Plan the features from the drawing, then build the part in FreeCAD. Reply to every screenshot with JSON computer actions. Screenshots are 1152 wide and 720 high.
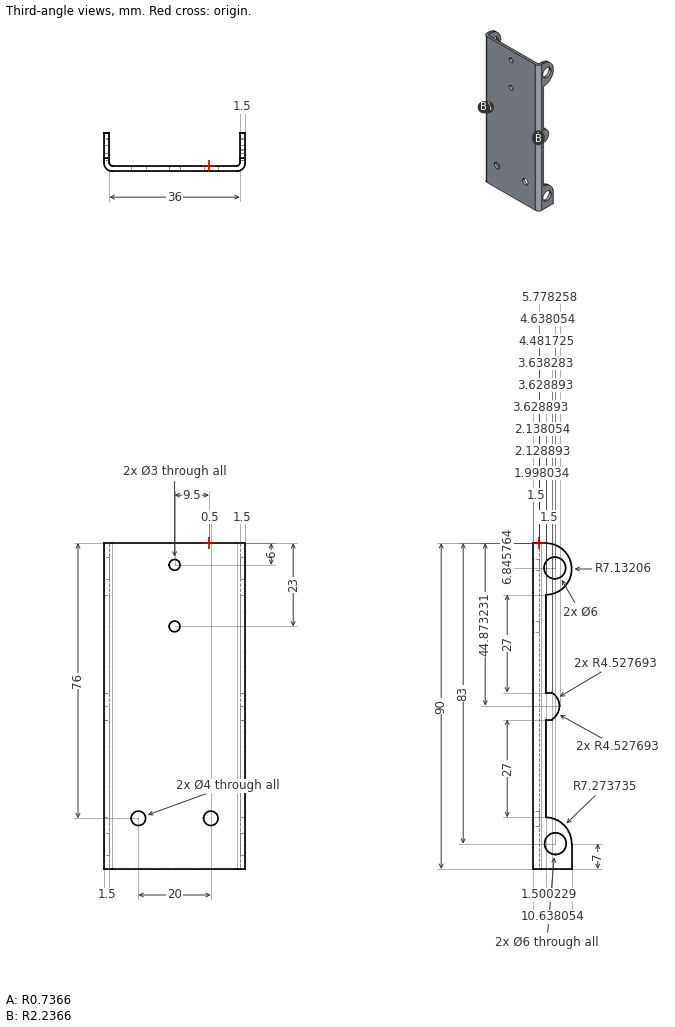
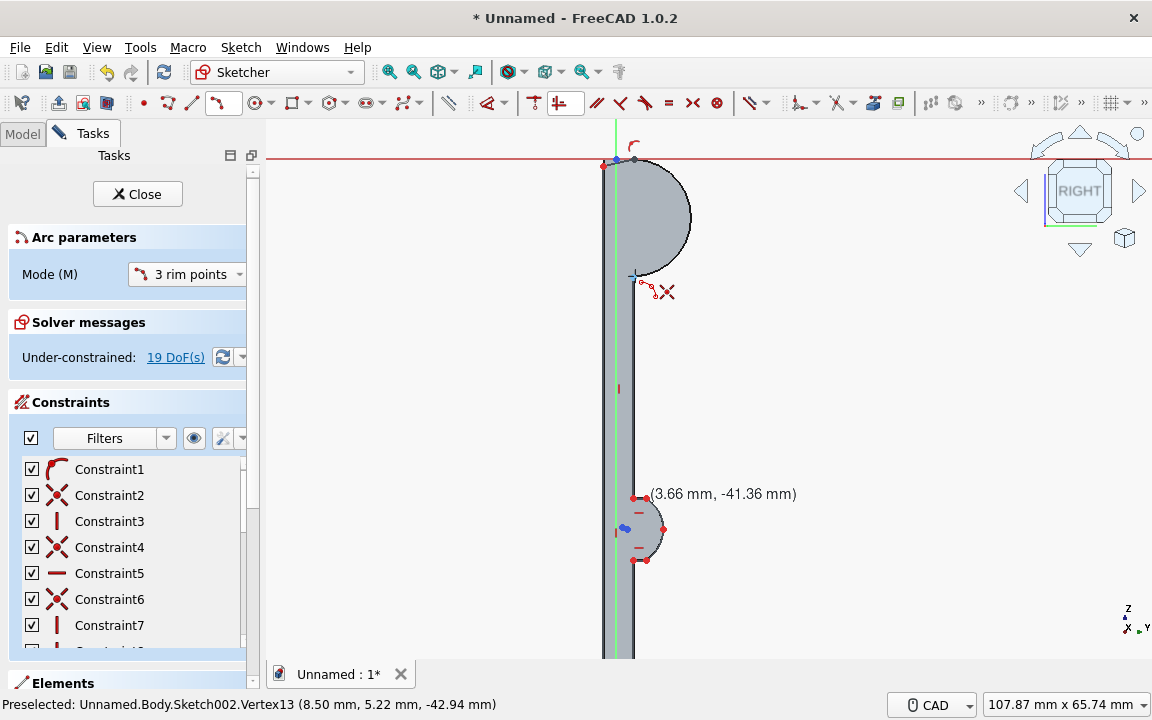
{"action": "left_click", "coordinate": [633, 278]}
{"action": "left_click", "coordinate": [634, 159]}
{"action": "left_click", "coordinate": [691, 218]}
{"action": "key", "text": "Escape"}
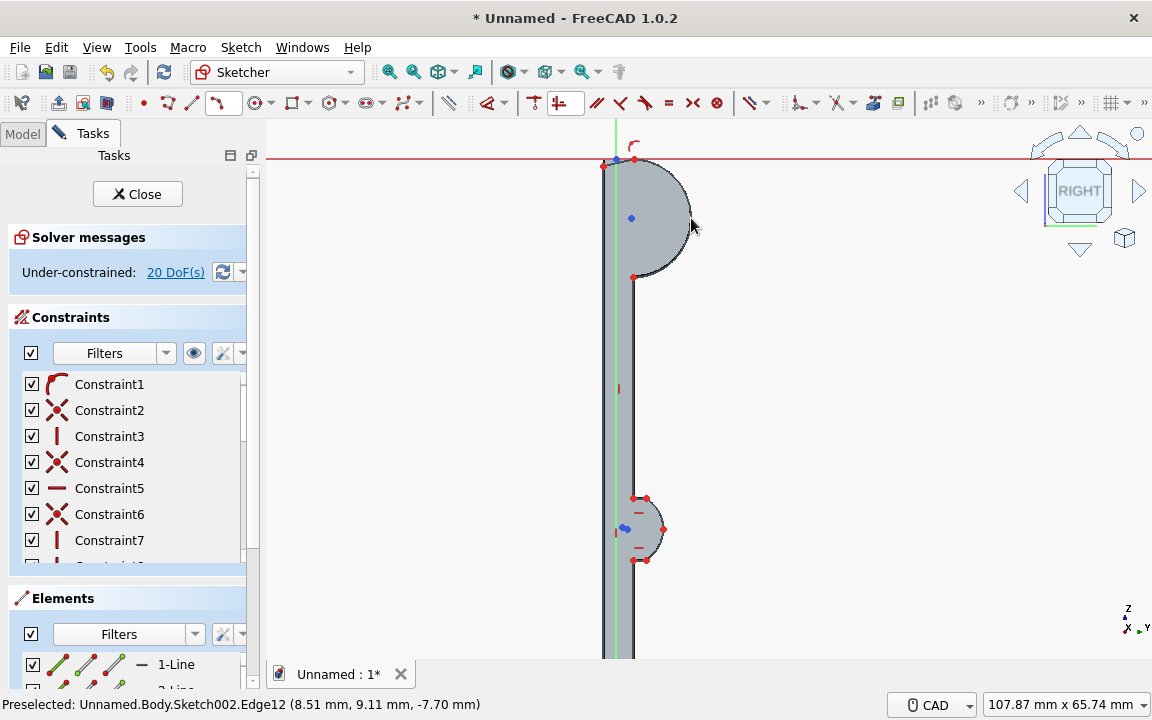
{"action": "scroll", "coordinate": [635, 275], "scroll_direction": "down", "scroll_amount": 4}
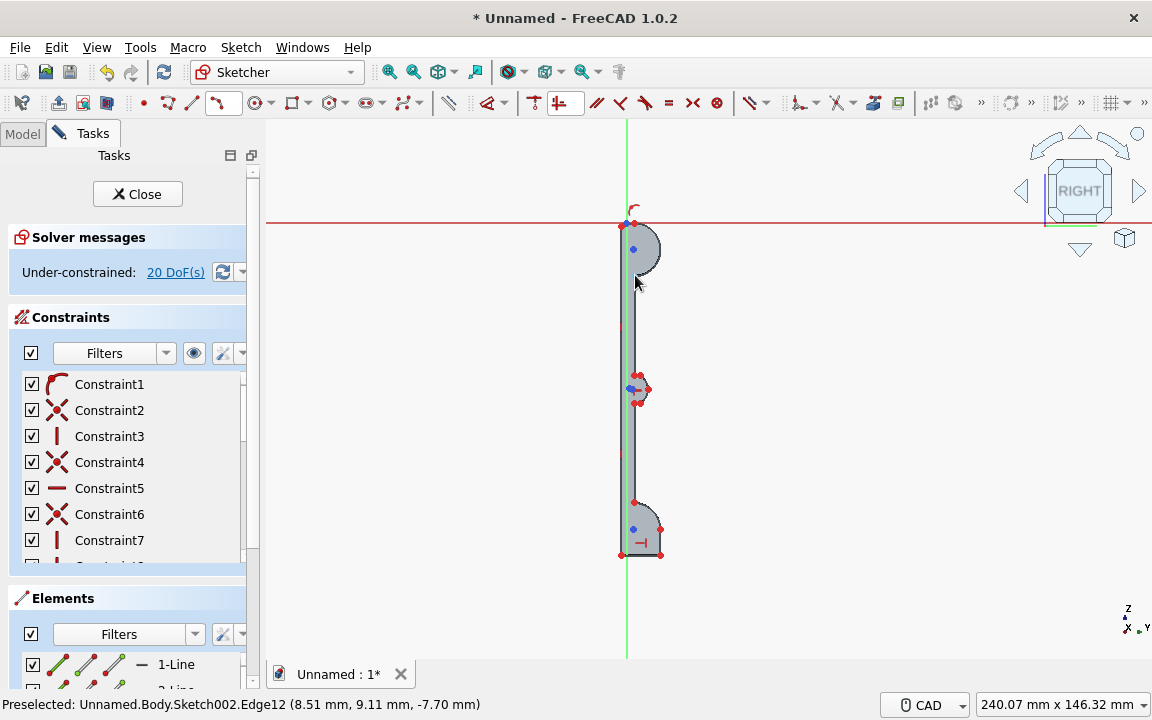
{"action": "scroll", "coordinate": [660, 548], "scroll_direction": "up", "scroll_amount": 3}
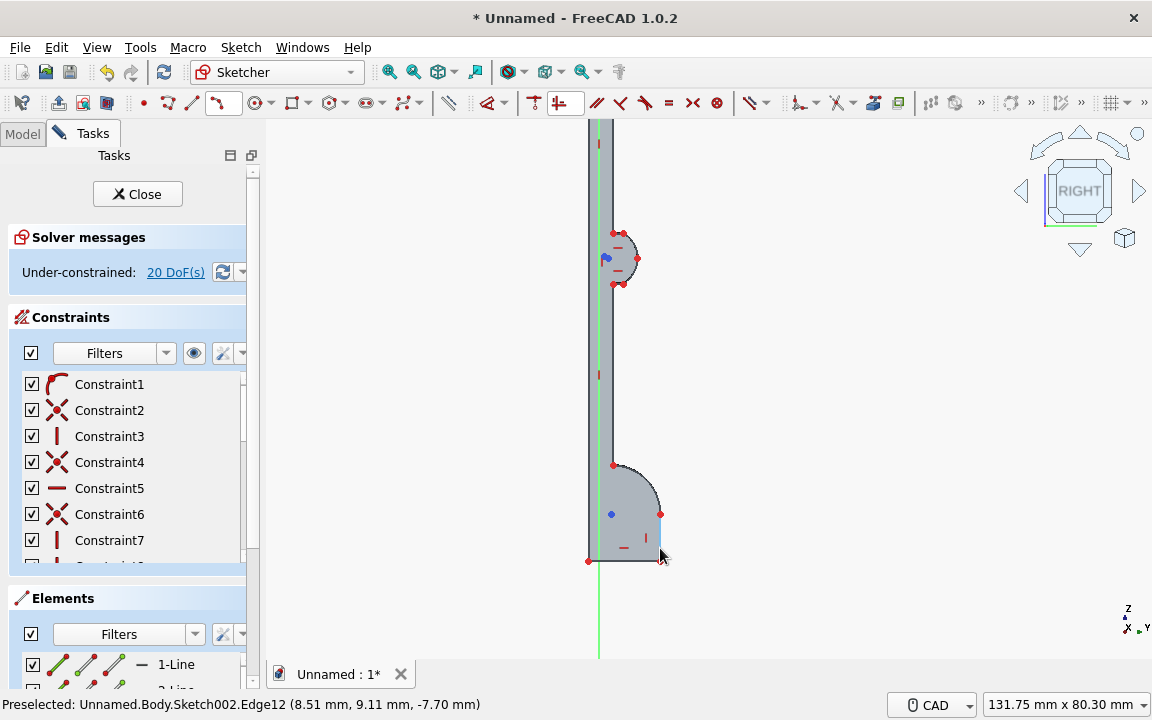
{"action": "left_click", "coordinate": [660, 547]}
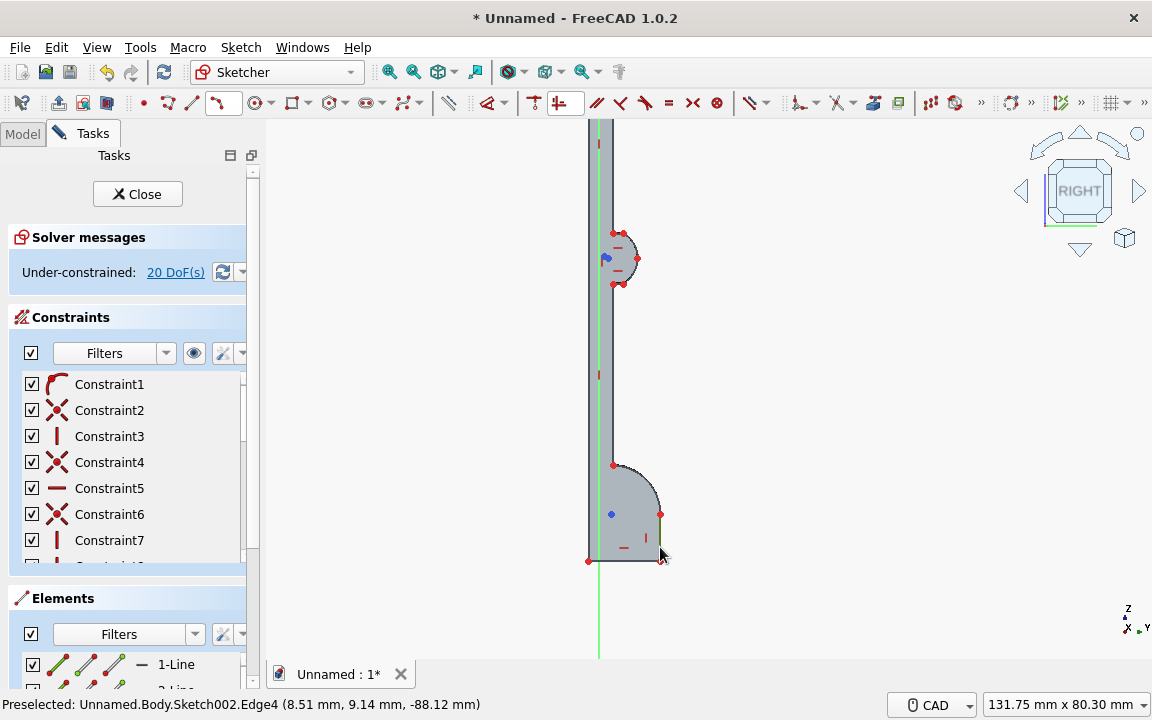
{"action": "left_click", "coordinate": [655, 492]}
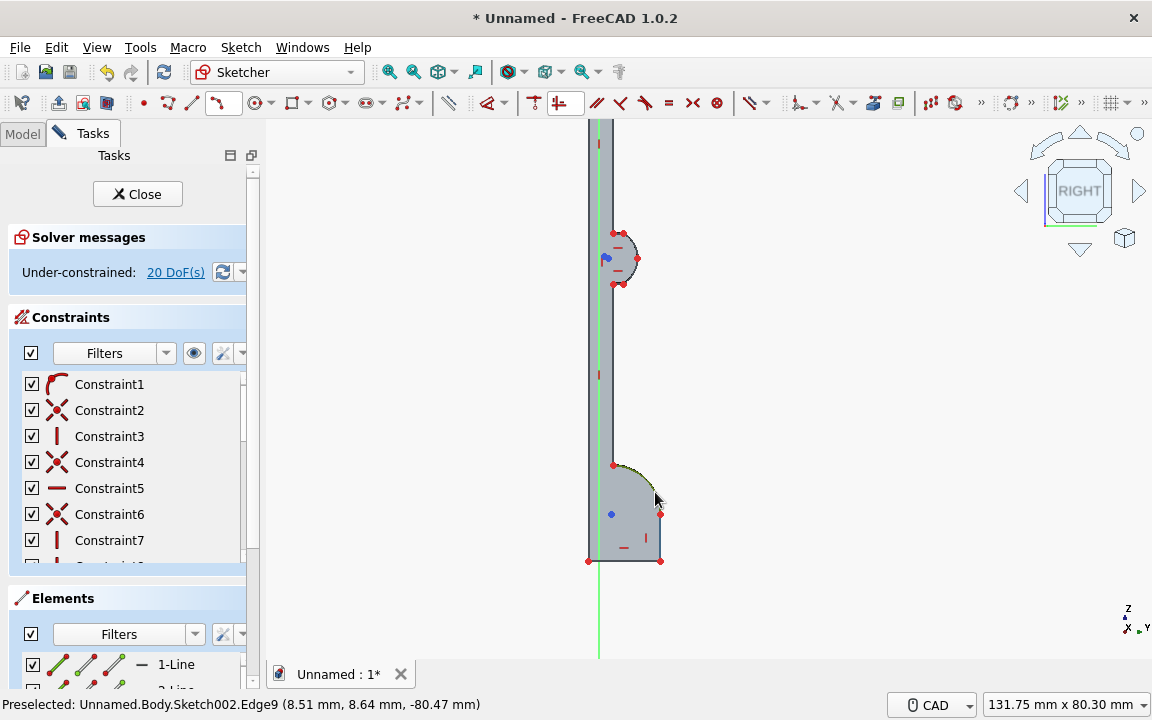
{"action": "key", "text": "t"}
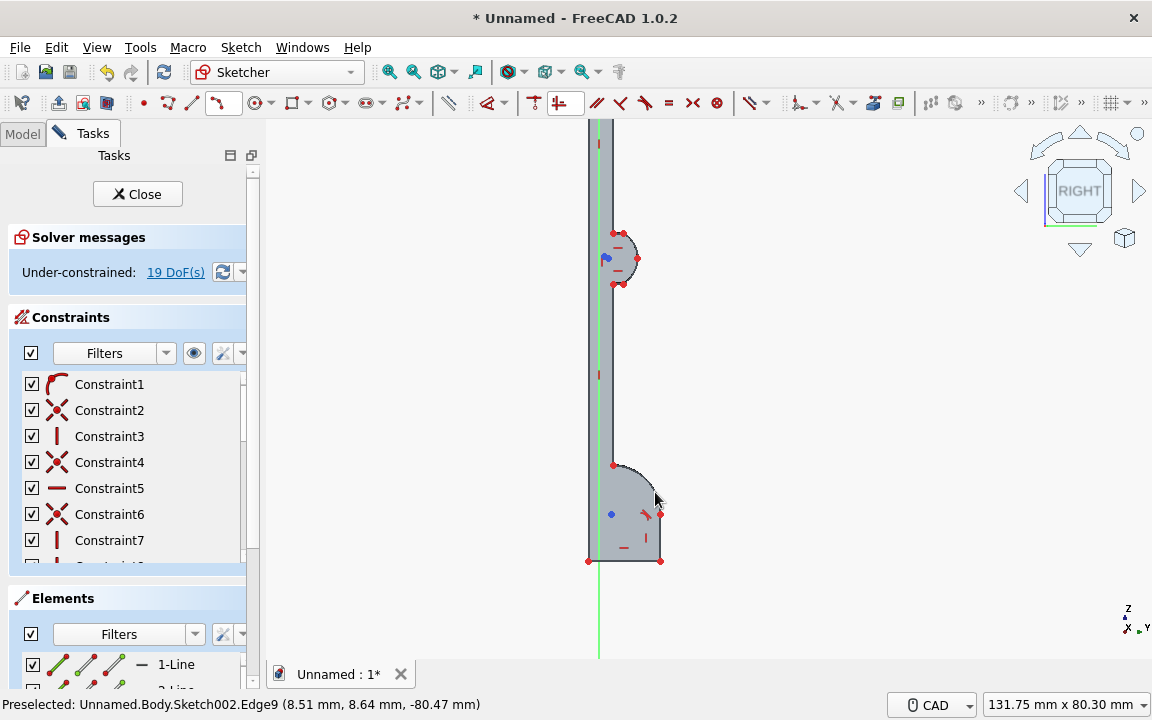
{"action": "scroll", "coordinate": [660, 548], "scroll_direction": "down", "scroll_amount": 3}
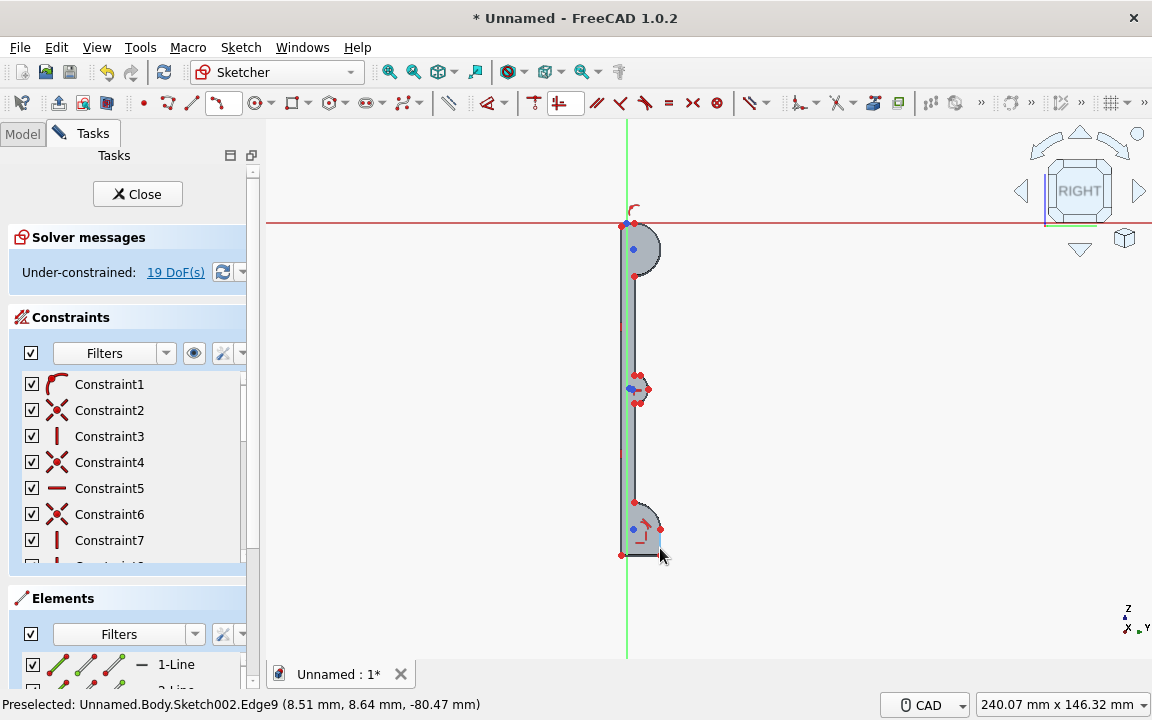
{"action": "scroll", "coordinate": [627, 225], "scroll_direction": "up", "scroll_amount": 5}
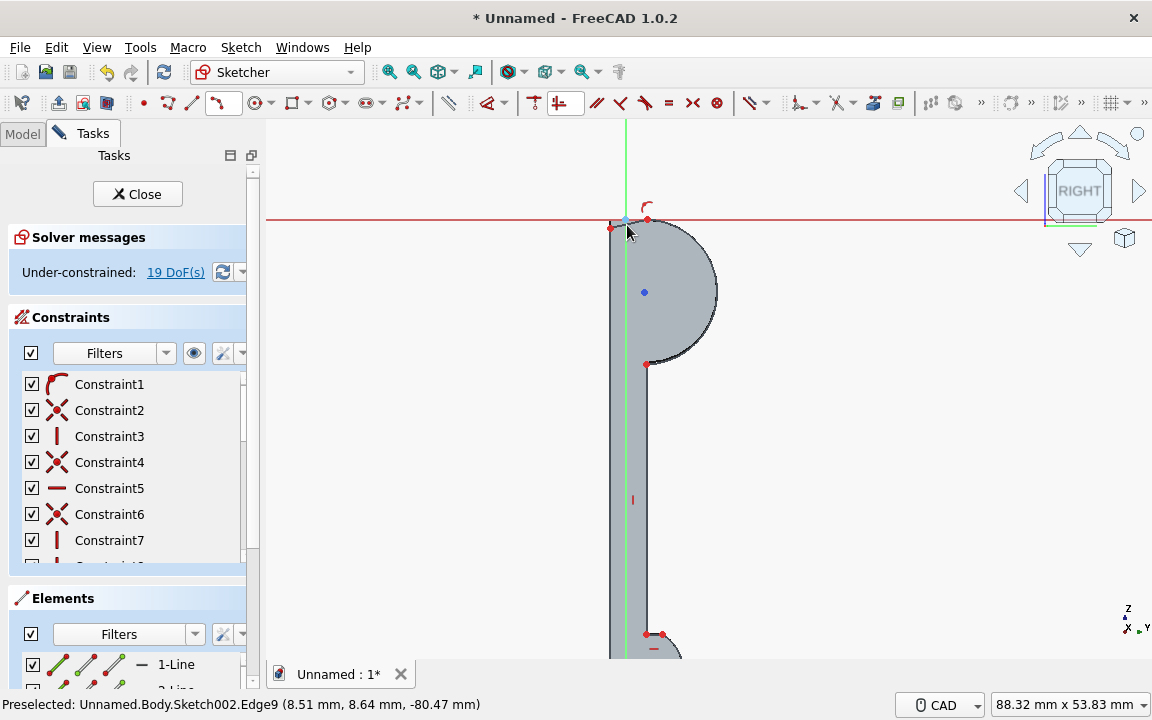
{"action": "left_click", "coordinate": [625, 225]}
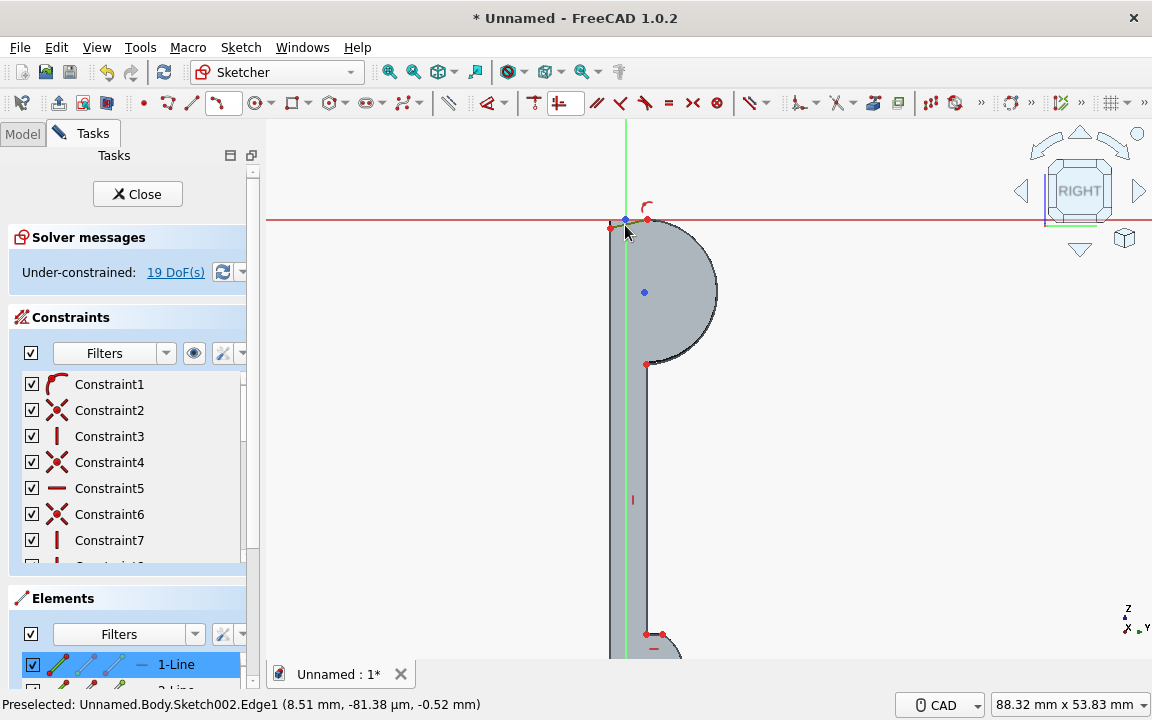
{"action": "key", "text": "h"}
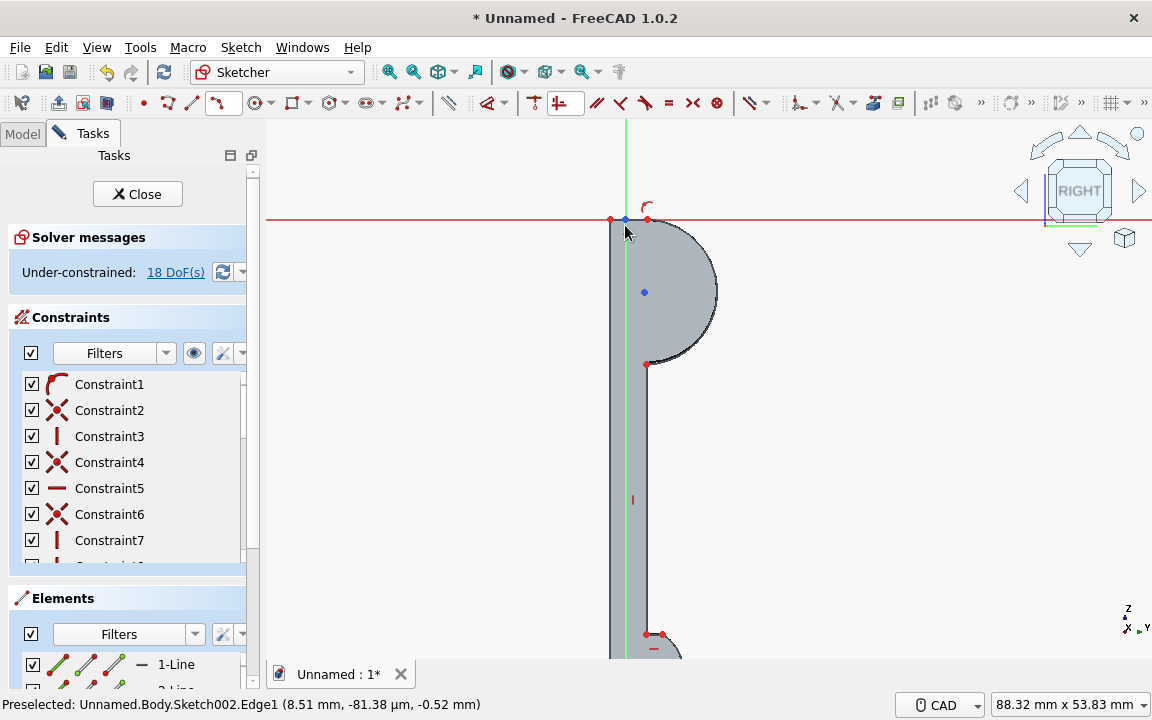
{"action": "scroll", "coordinate": [627, 225], "scroll_direction": "down", "scroll_amount": 5}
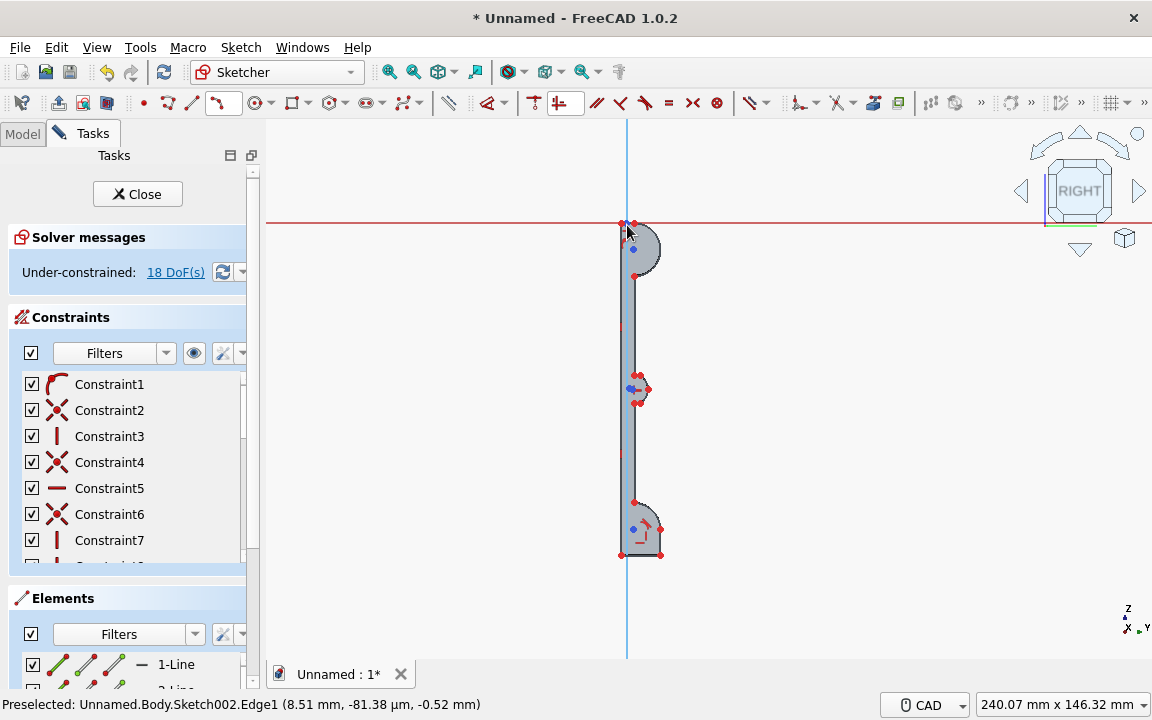
{"action": "scroll", "coordinate": [644, 400], "scroll_direction": "up", "scroll_amount": 6}